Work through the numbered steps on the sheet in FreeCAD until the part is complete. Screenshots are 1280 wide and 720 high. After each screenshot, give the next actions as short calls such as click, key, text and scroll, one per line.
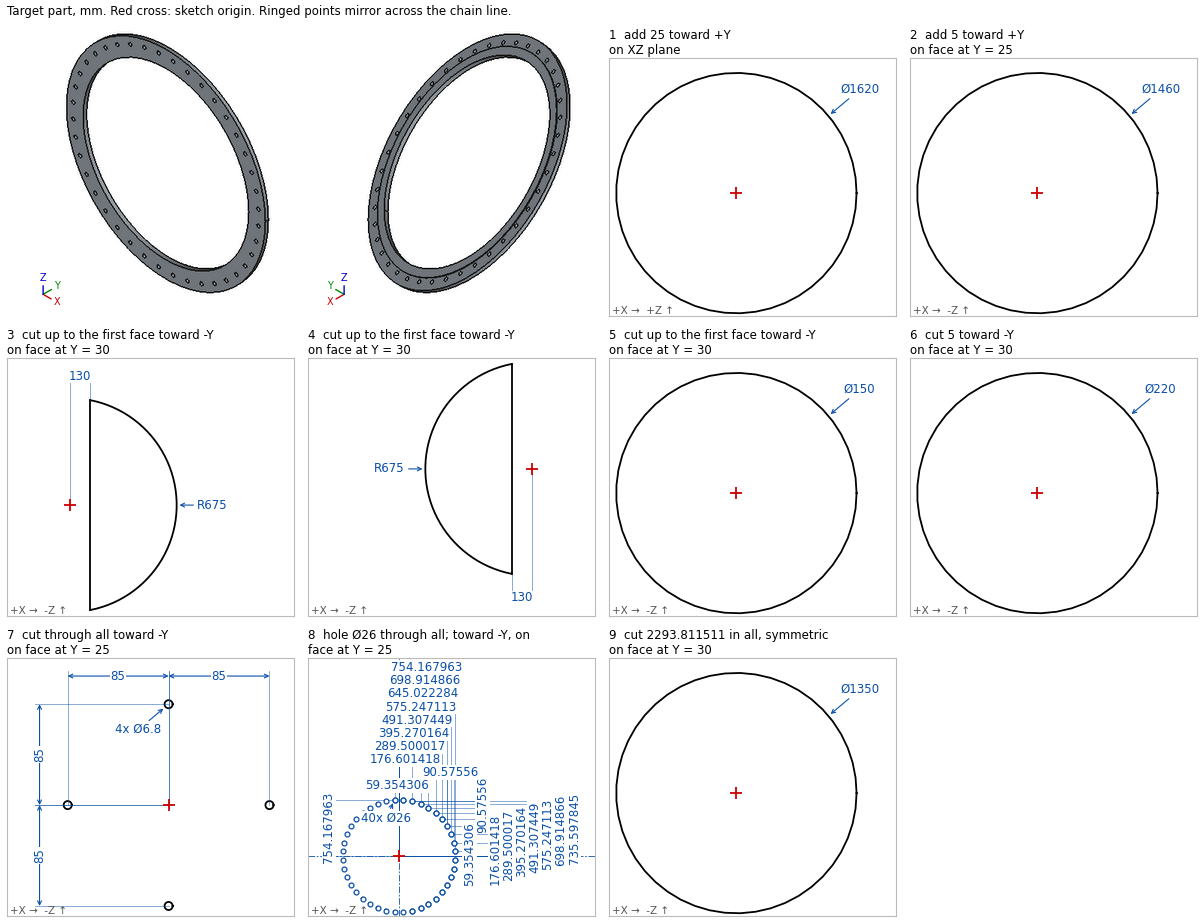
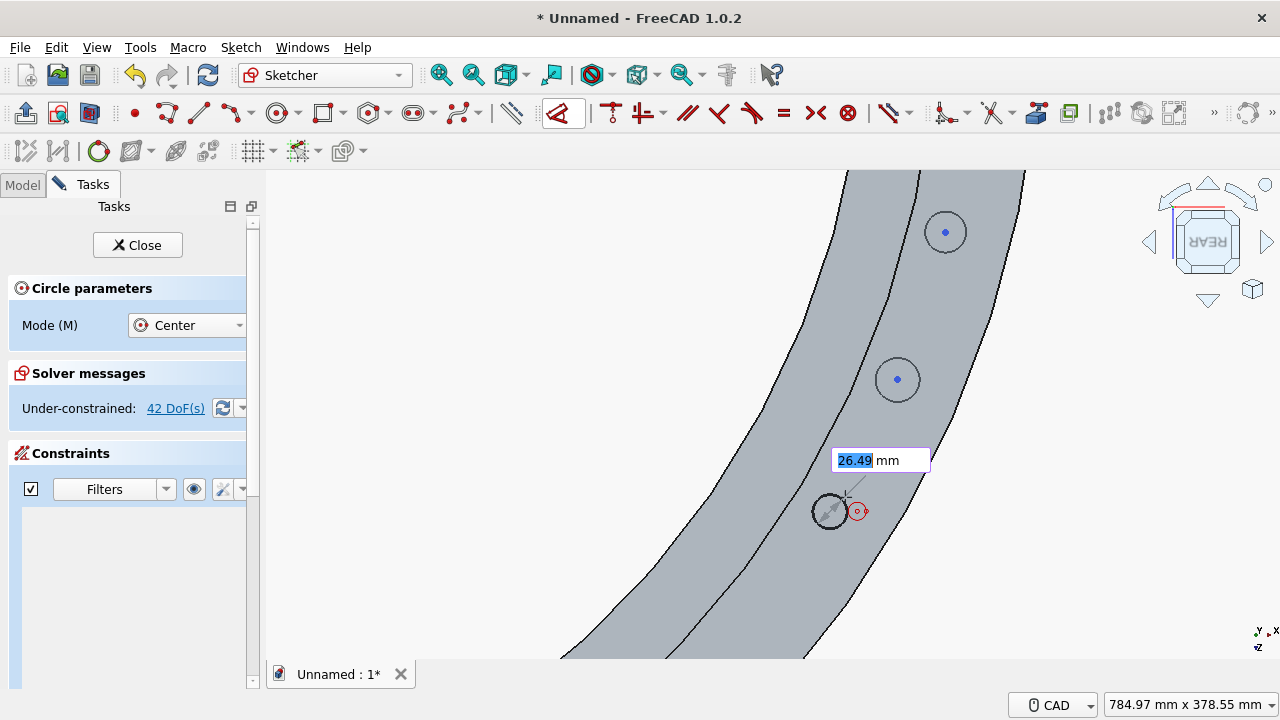
click(839, 496)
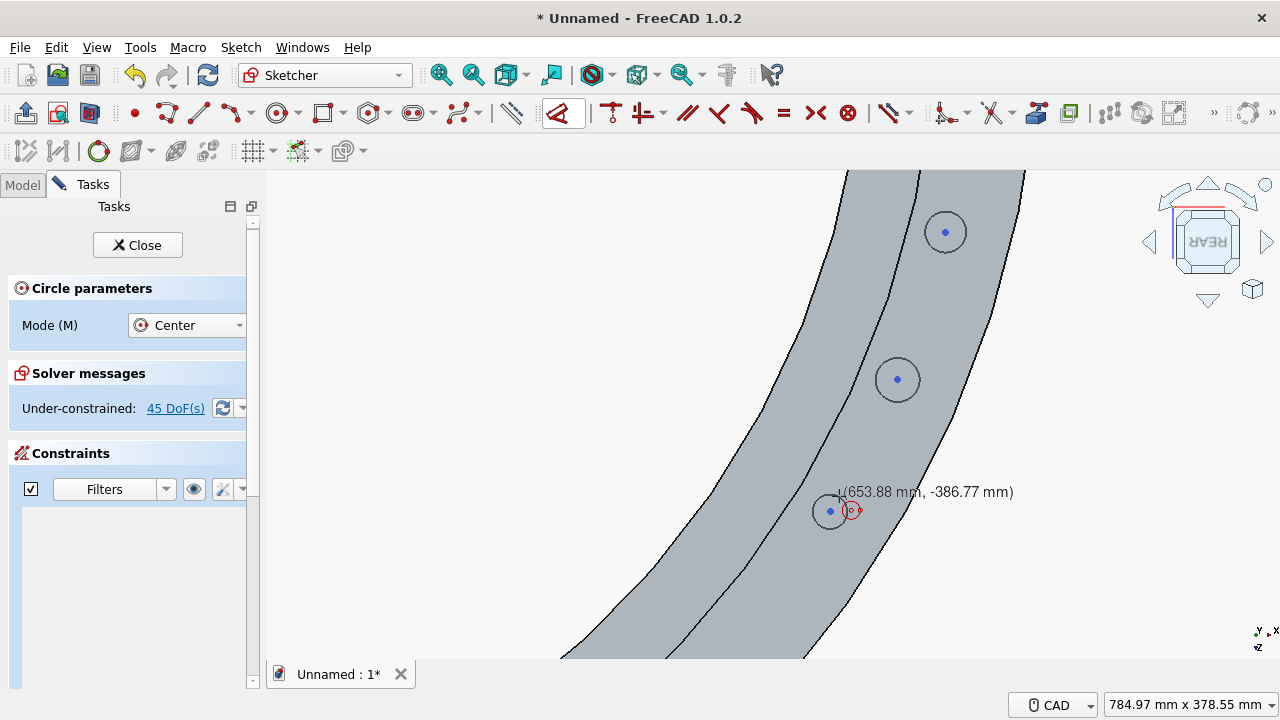
scroll(845, 497, down, 9)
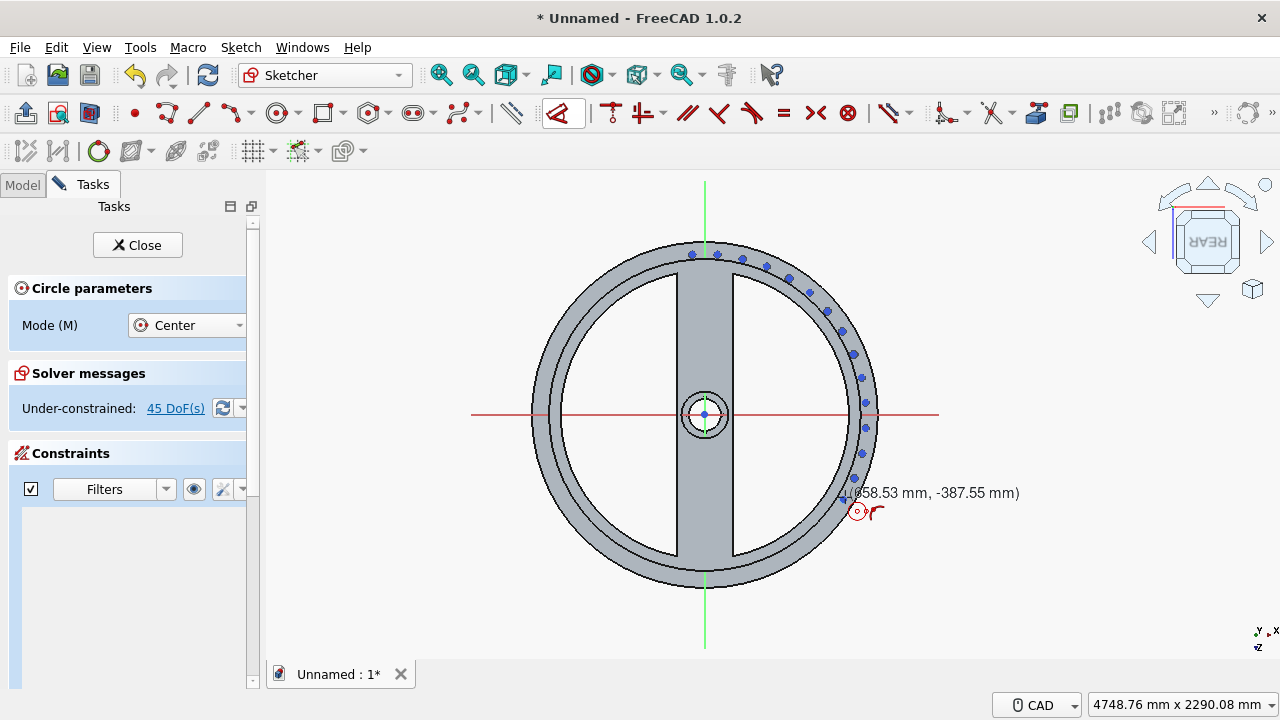
scroll(828, 520, up, 11)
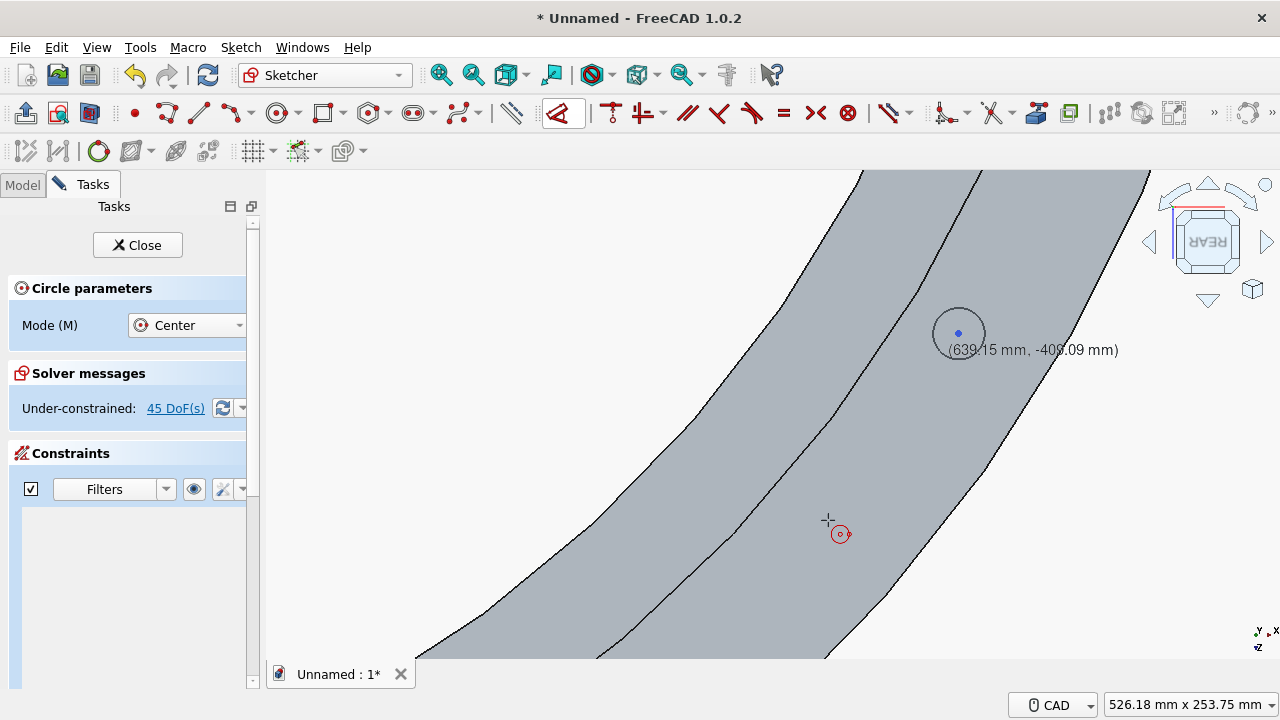
scroll(828, 520, down, 11)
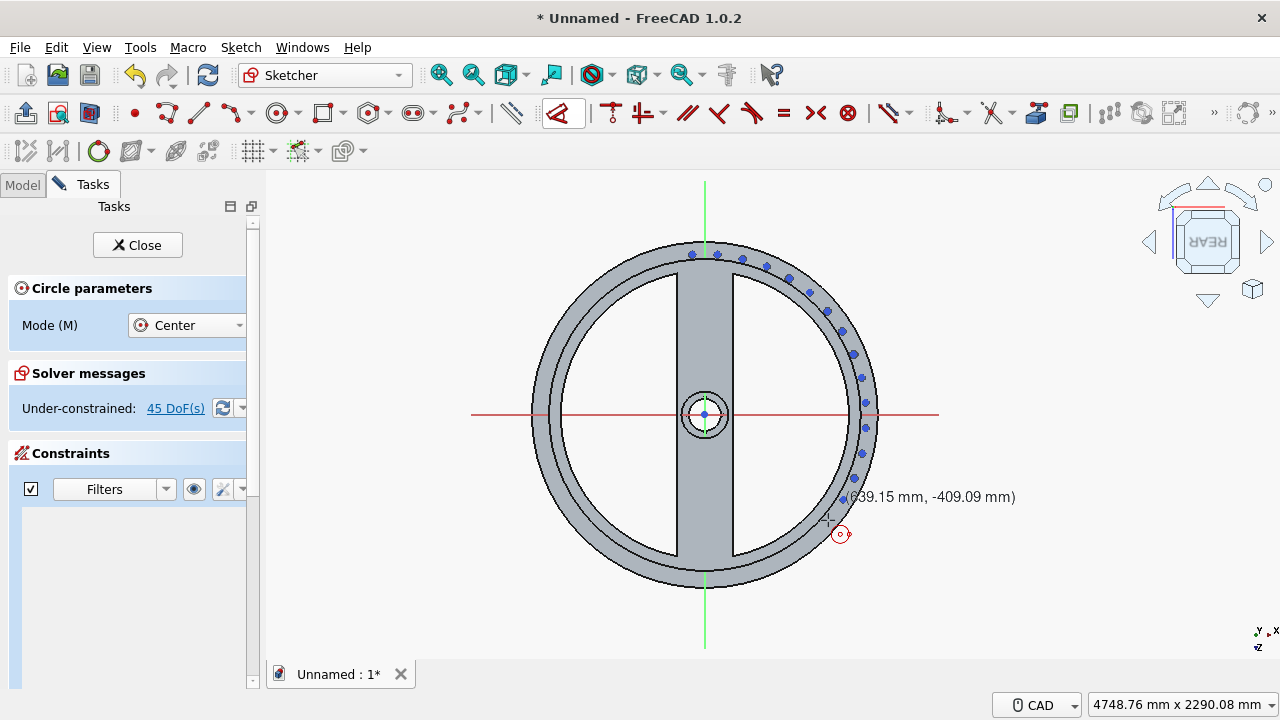
click(828, 520)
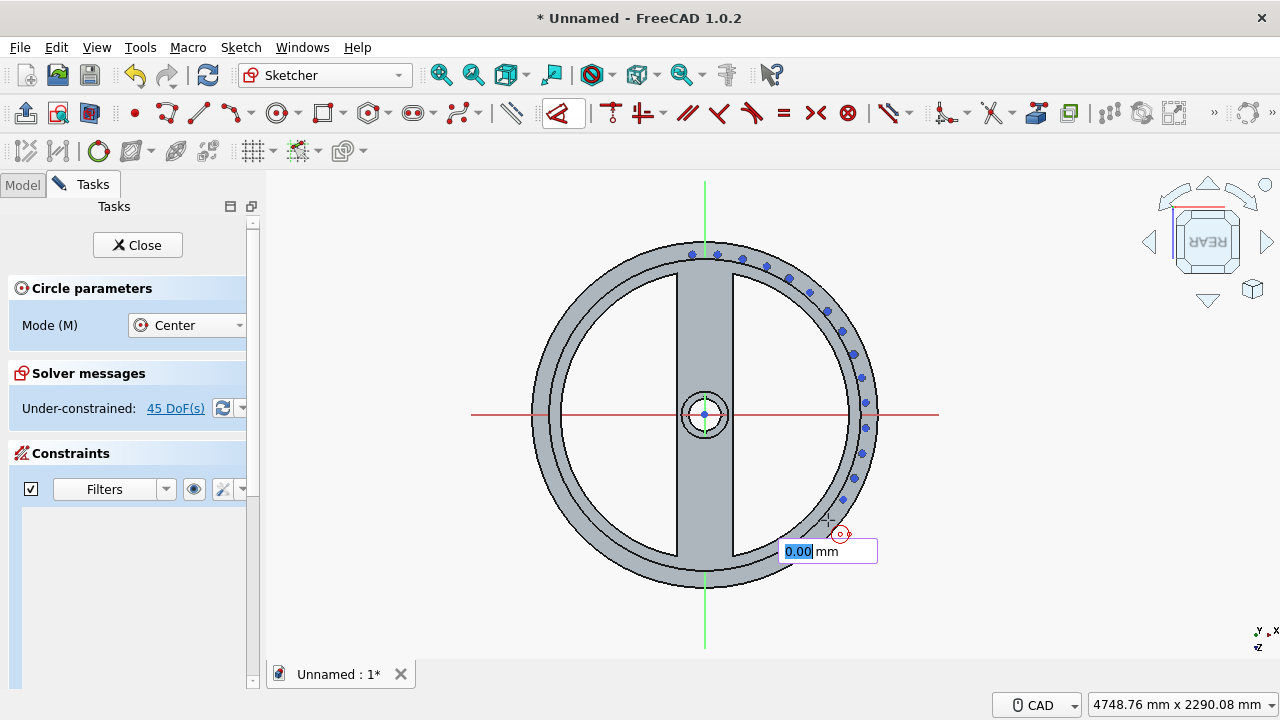
scroll(830, 518, up, 9)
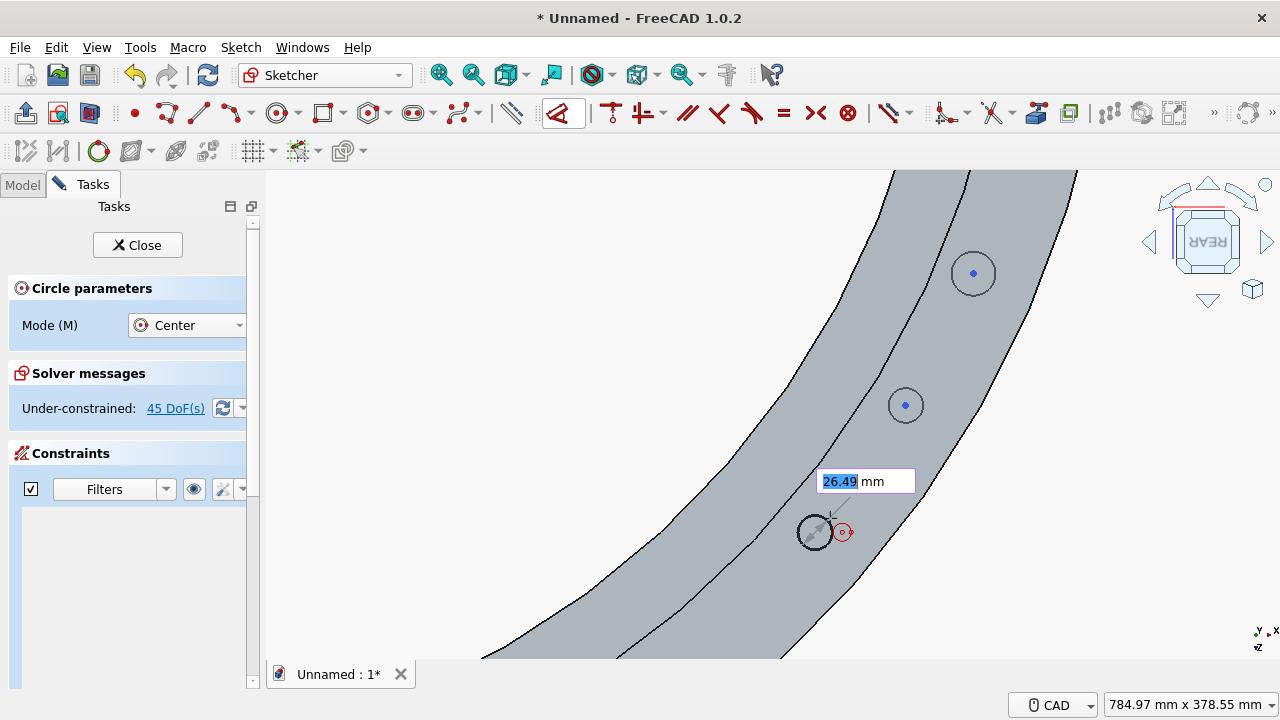
click(825, 514)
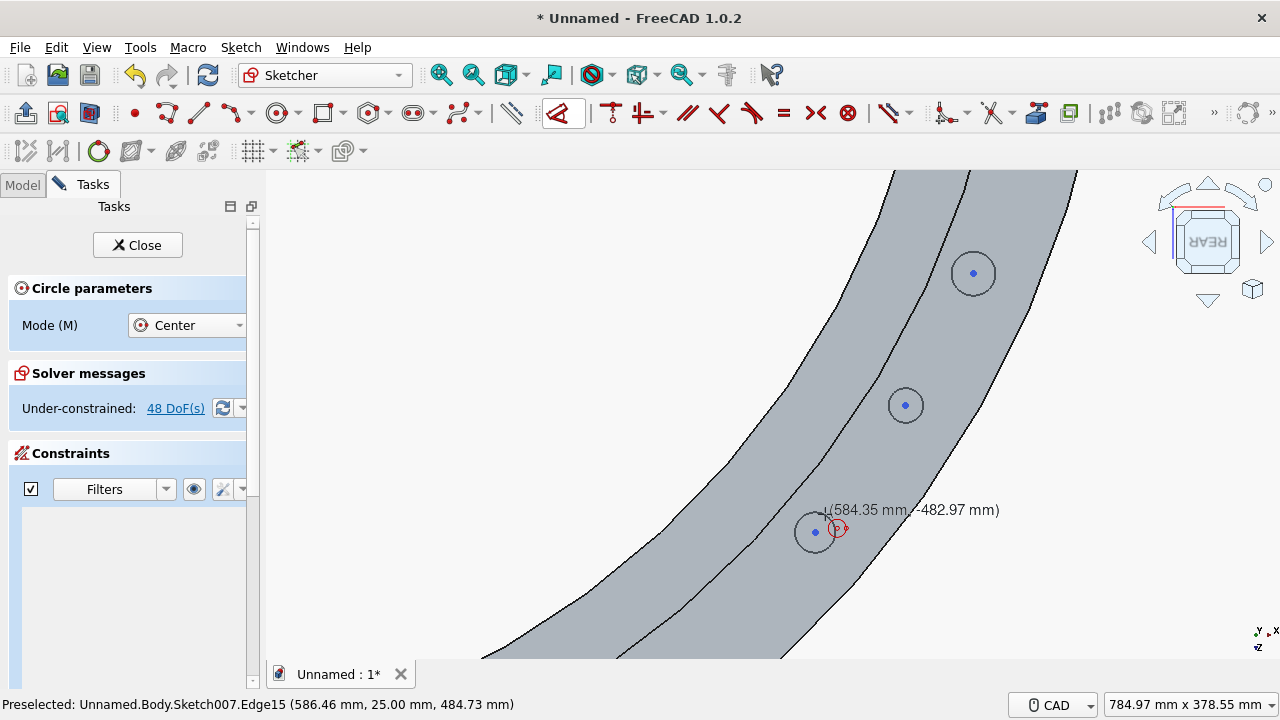
scroll(830, 518, down, 9)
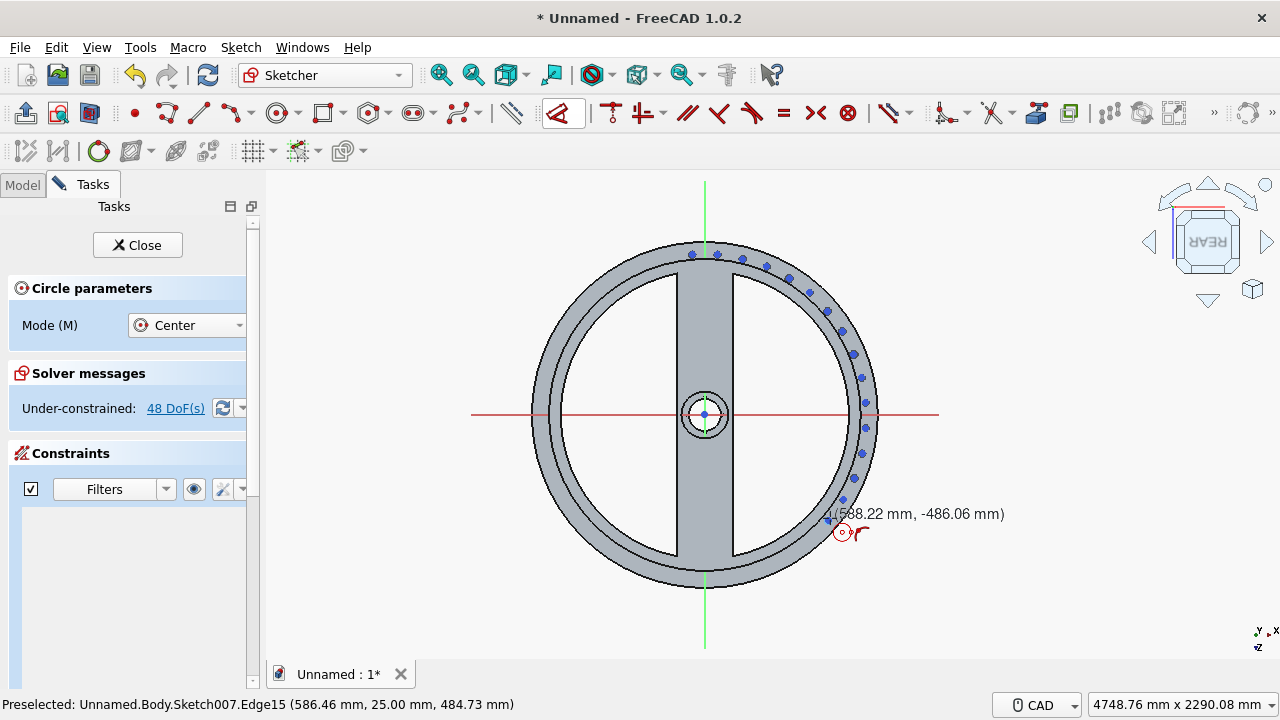
scroll(810, 538, up, 11)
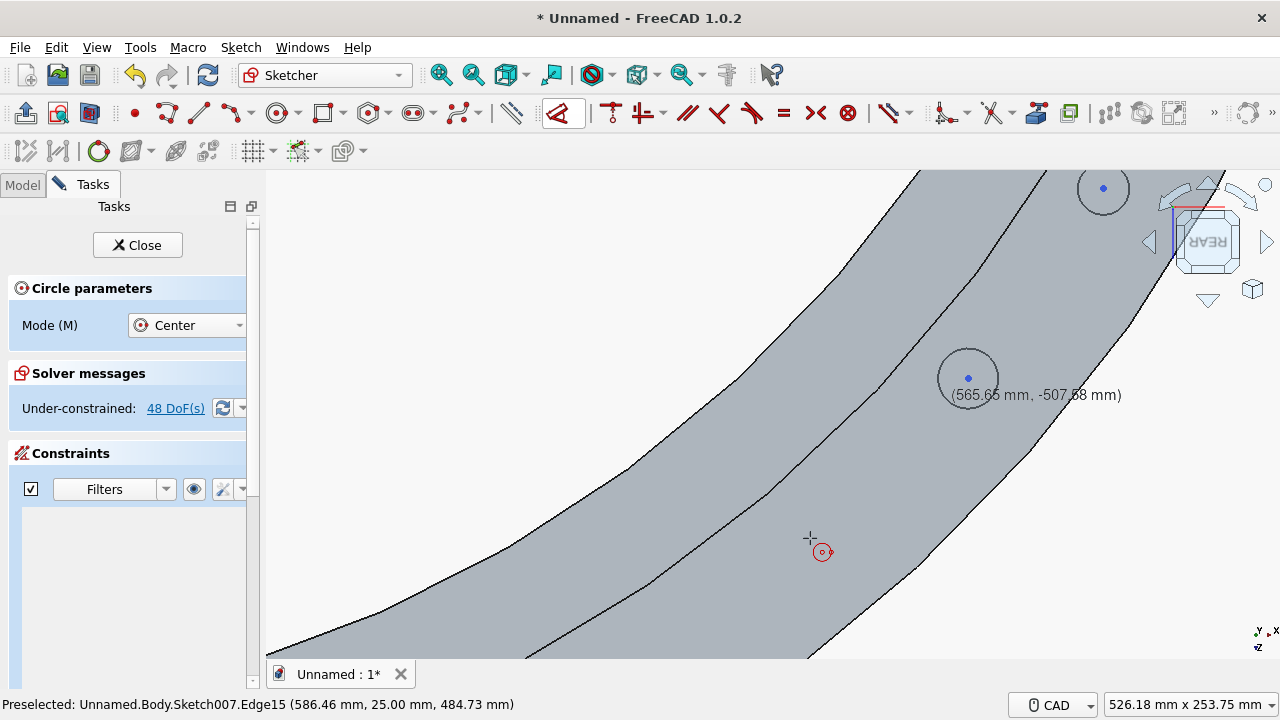
scroll(810, 538, down, 11)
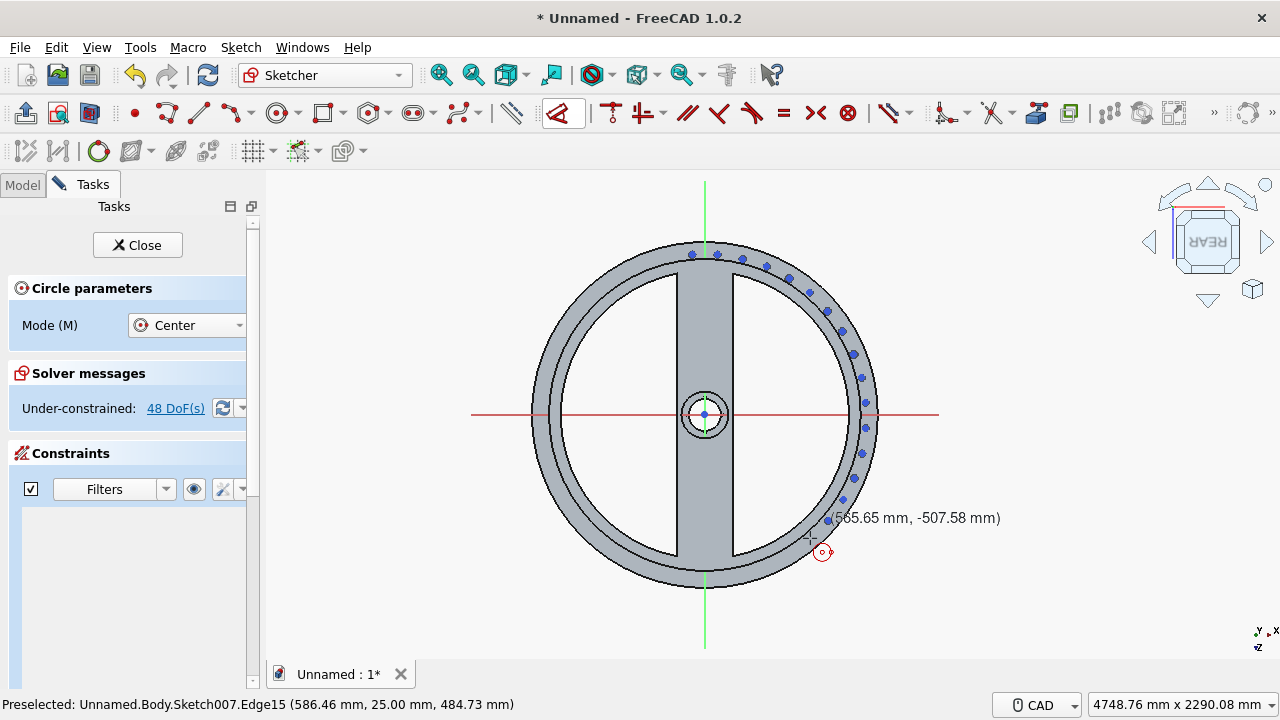
click(810, 538)